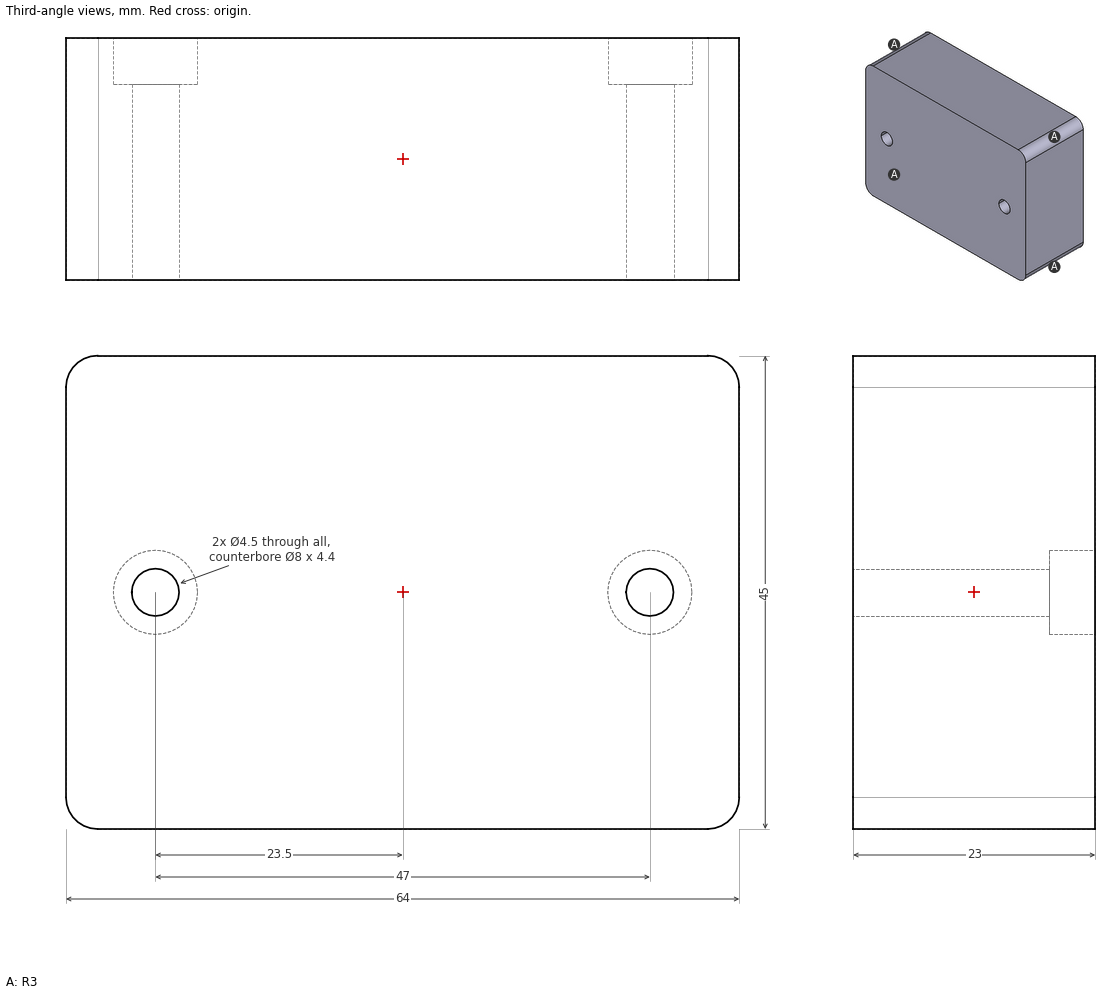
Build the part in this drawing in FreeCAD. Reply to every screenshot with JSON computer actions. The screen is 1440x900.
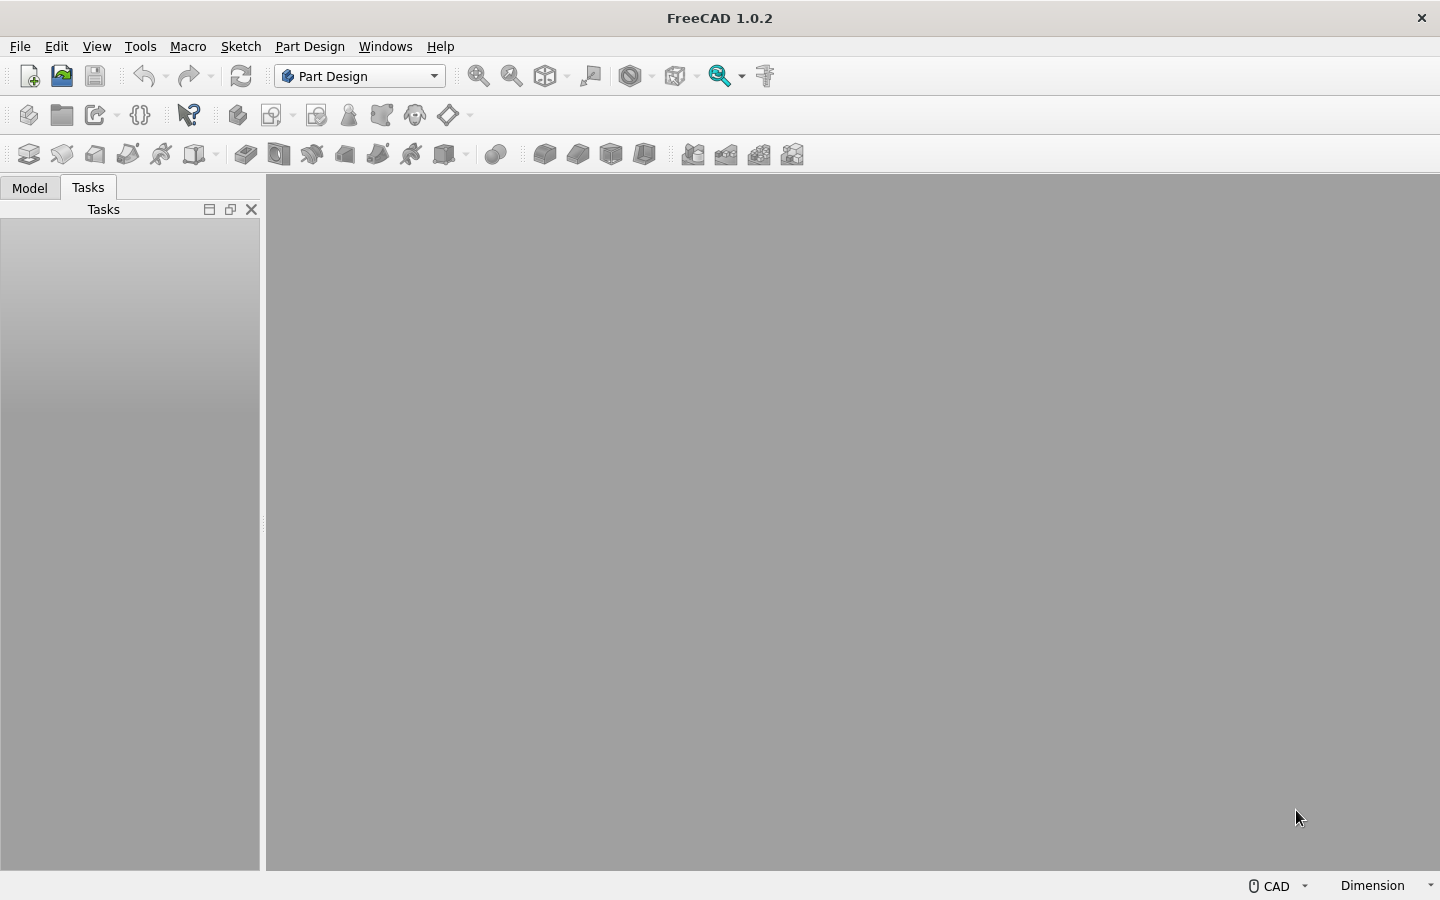
{"action": "left_click", "coordinate": [29, 76]}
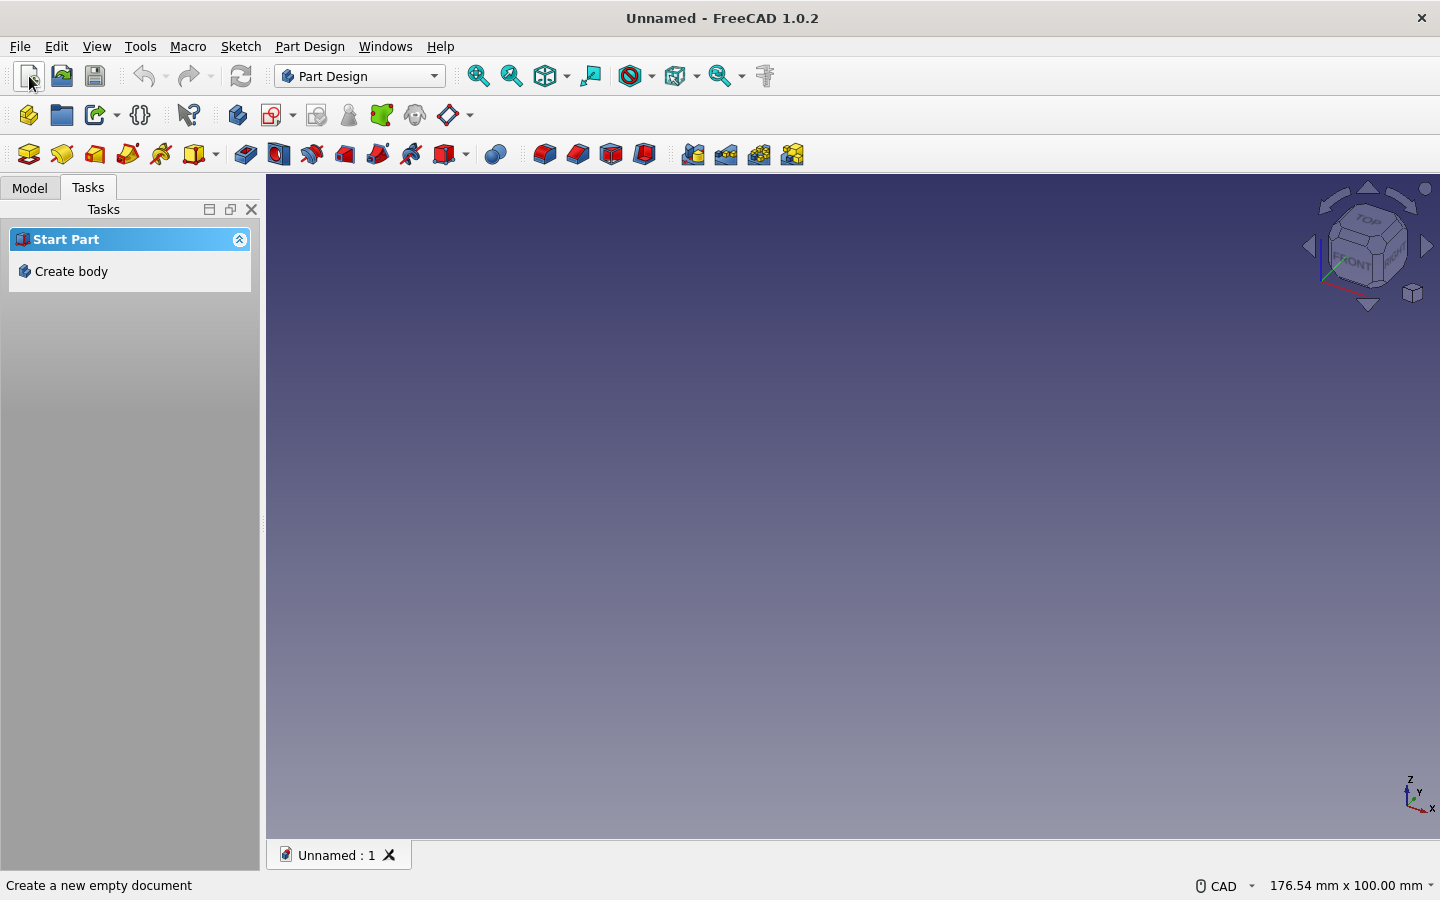
{"action": "left_click", "coordinate": [270, 116]}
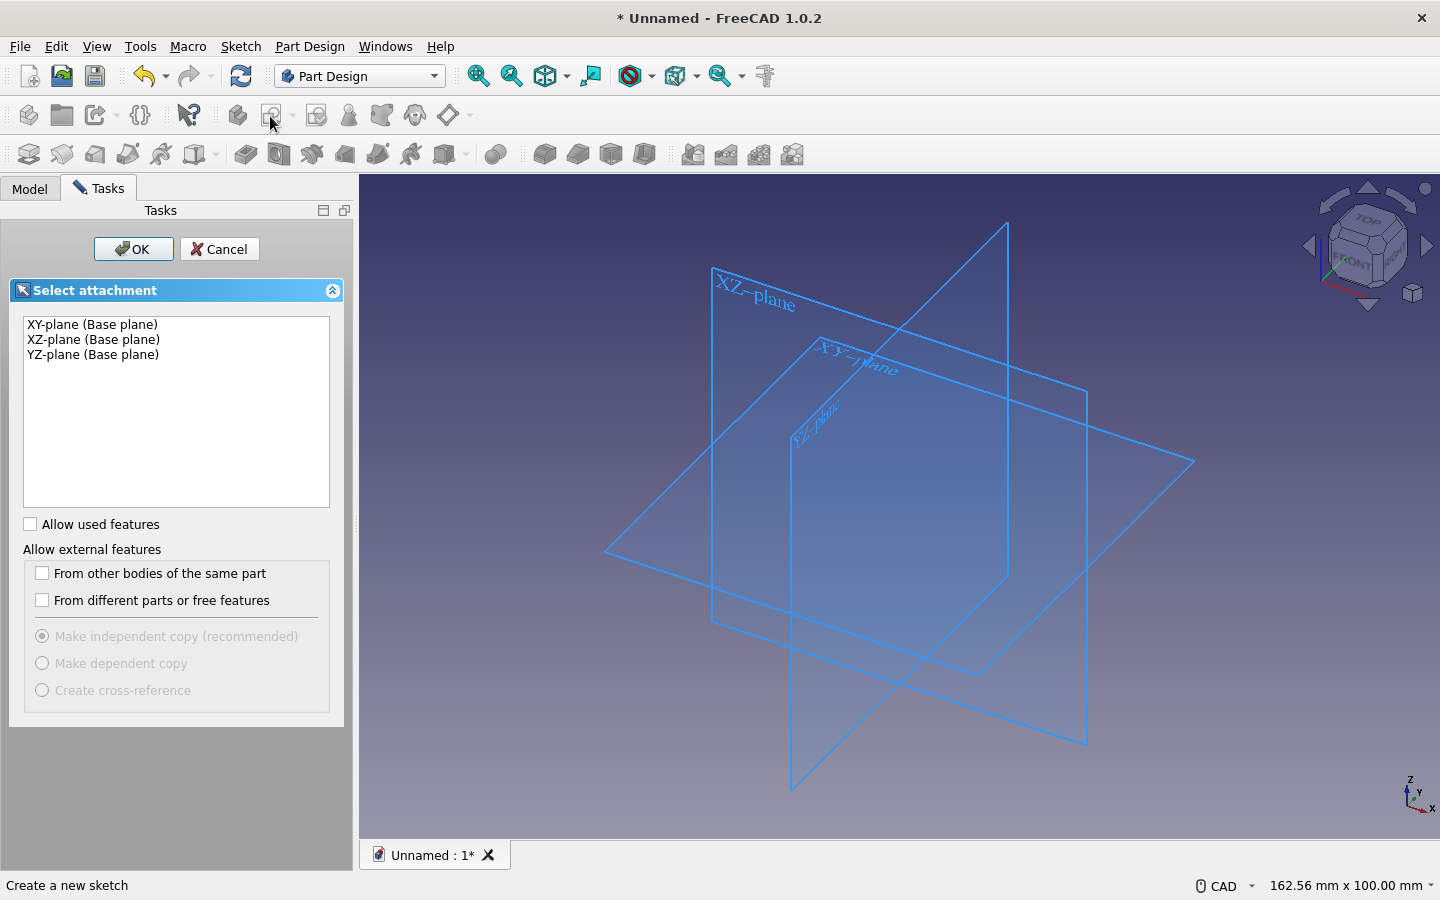
{"action": "left_click", "coordinate": [84, 340]}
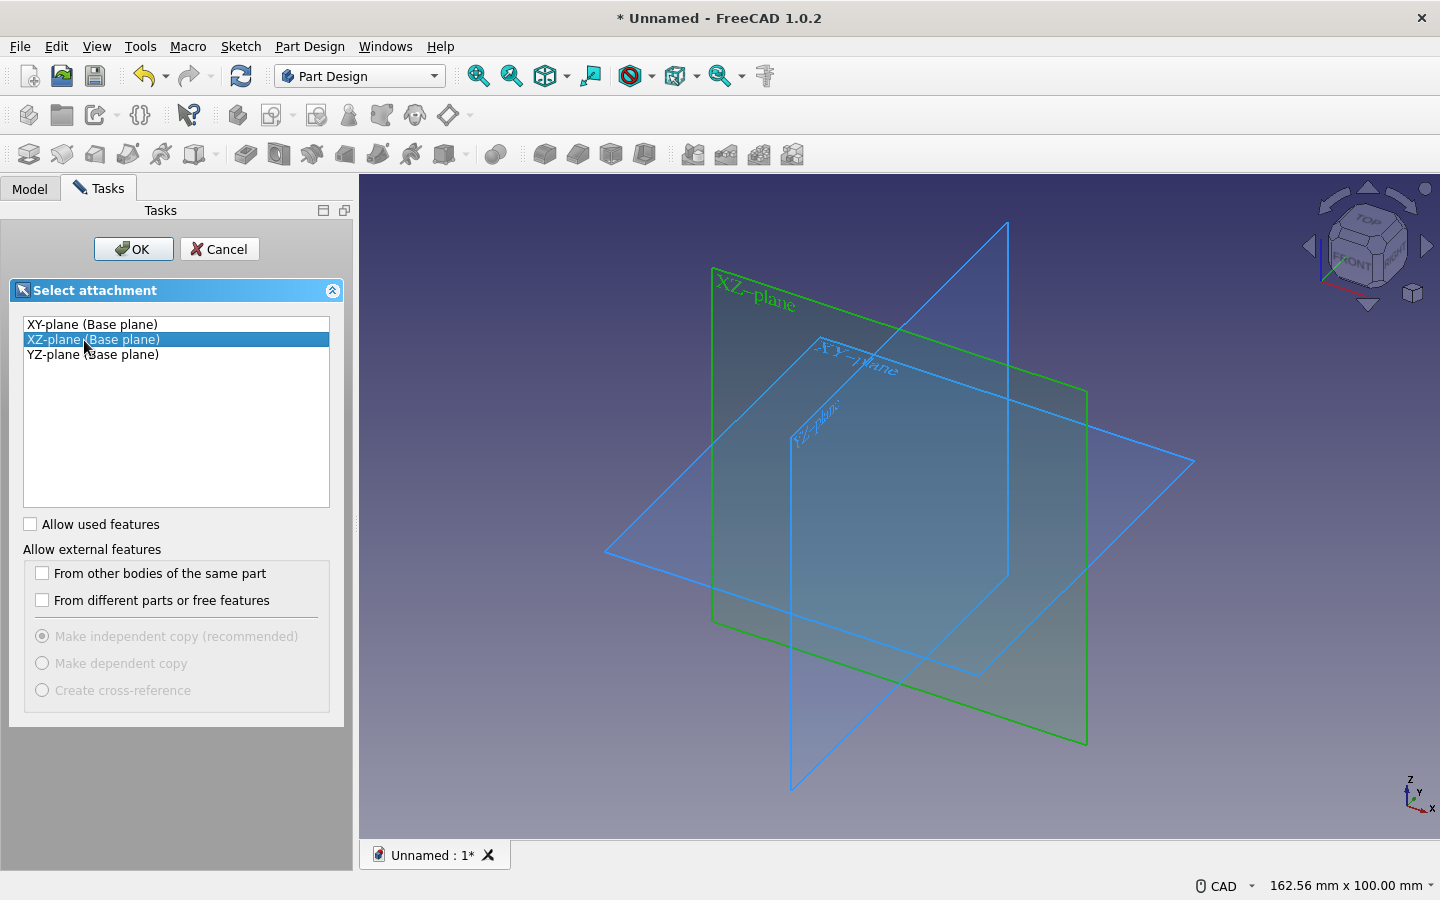
{"action": "left_click", "coordinate": [134, 249]}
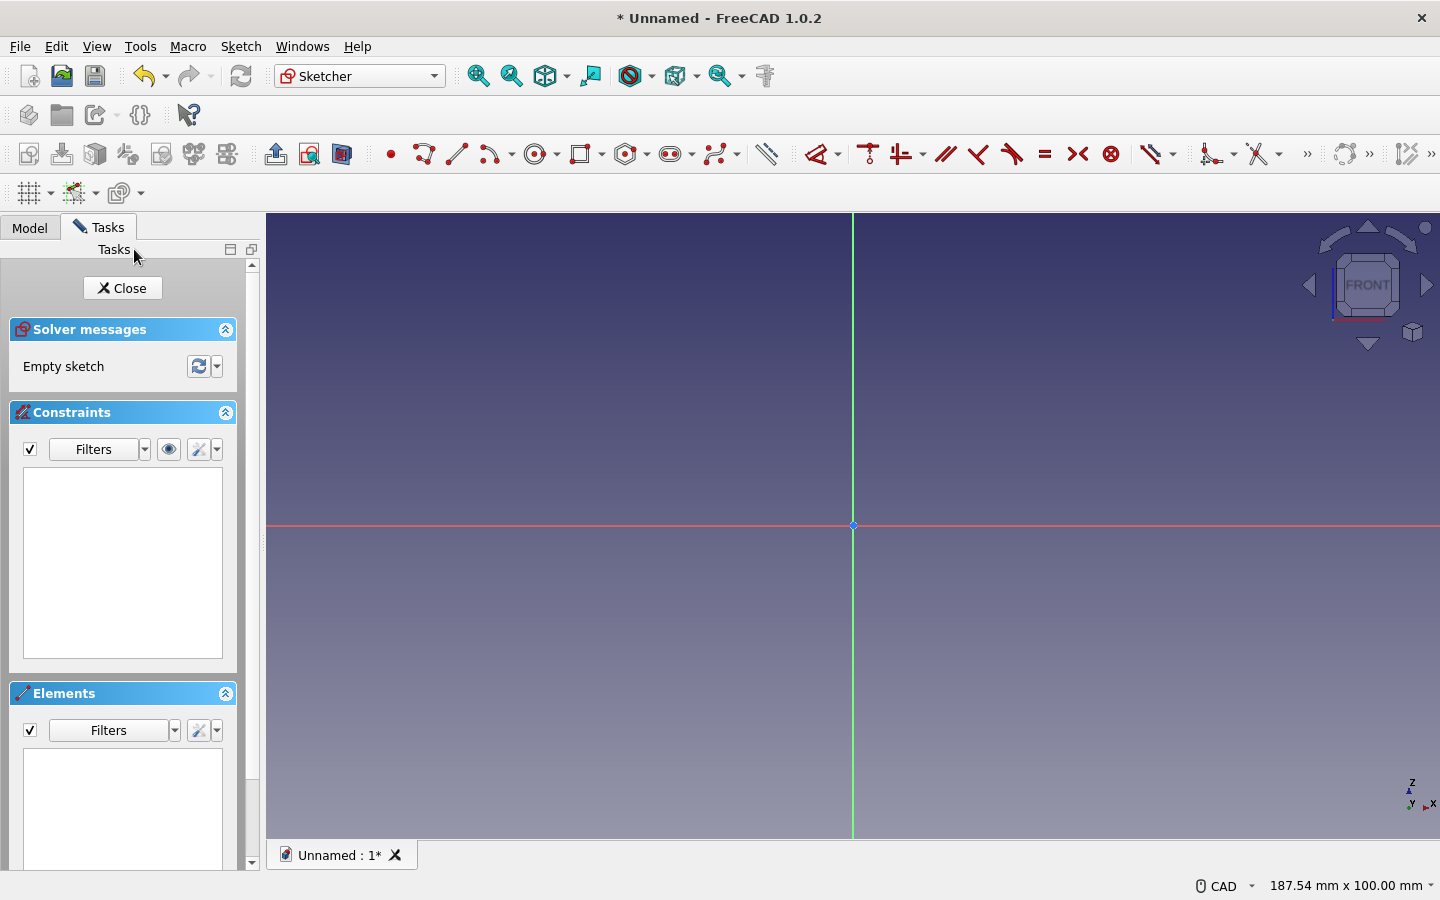
{"action": "scroll", "coordinate": [992, 526], "scroll_direction": "up", "scroll_amount": 2}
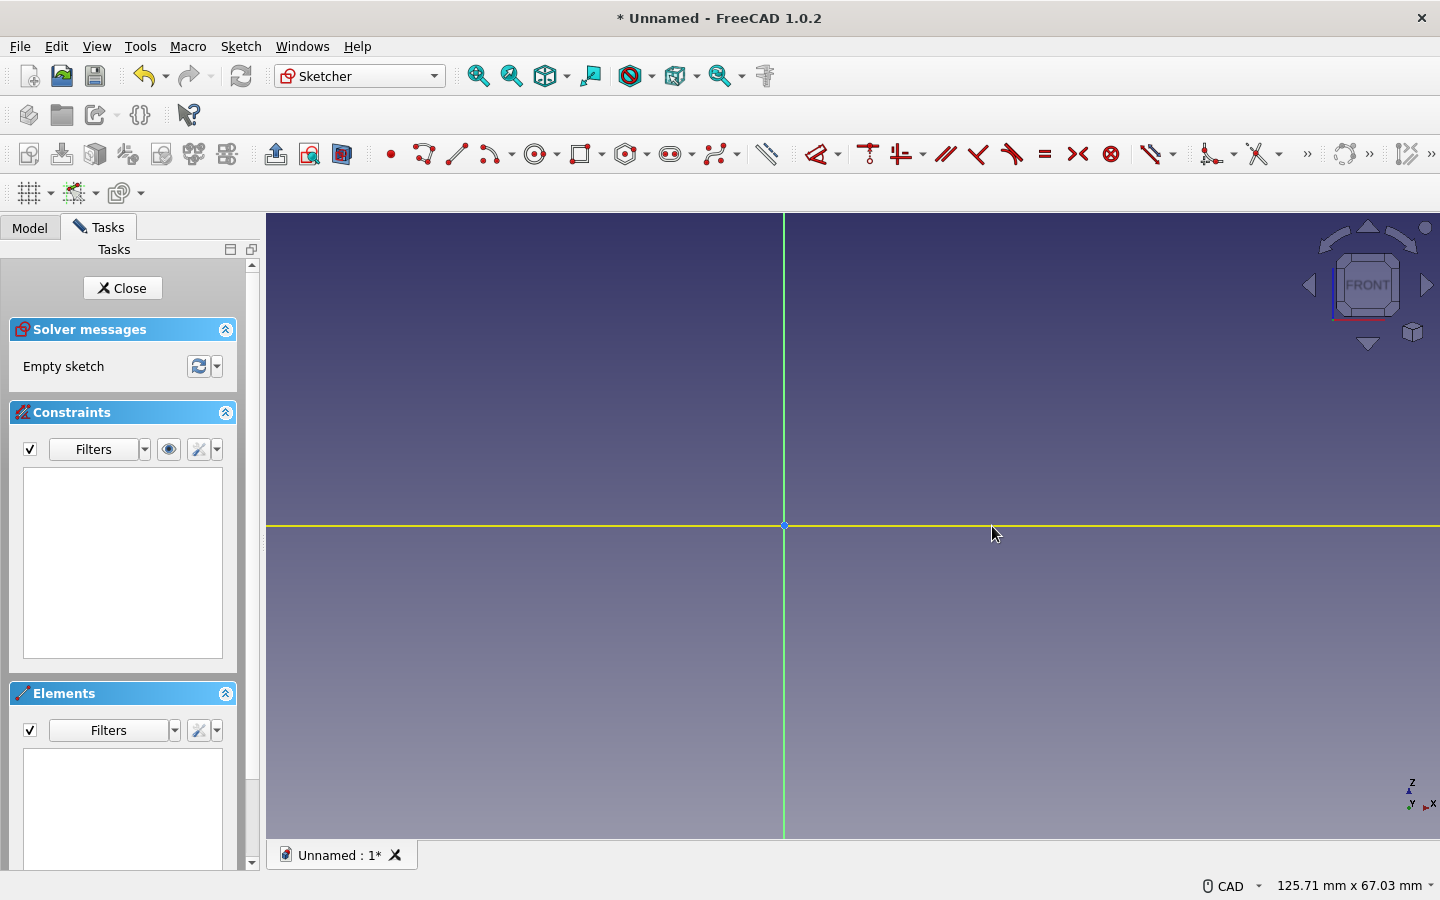
{"action": "left_click", "coordinate": [602, 154]}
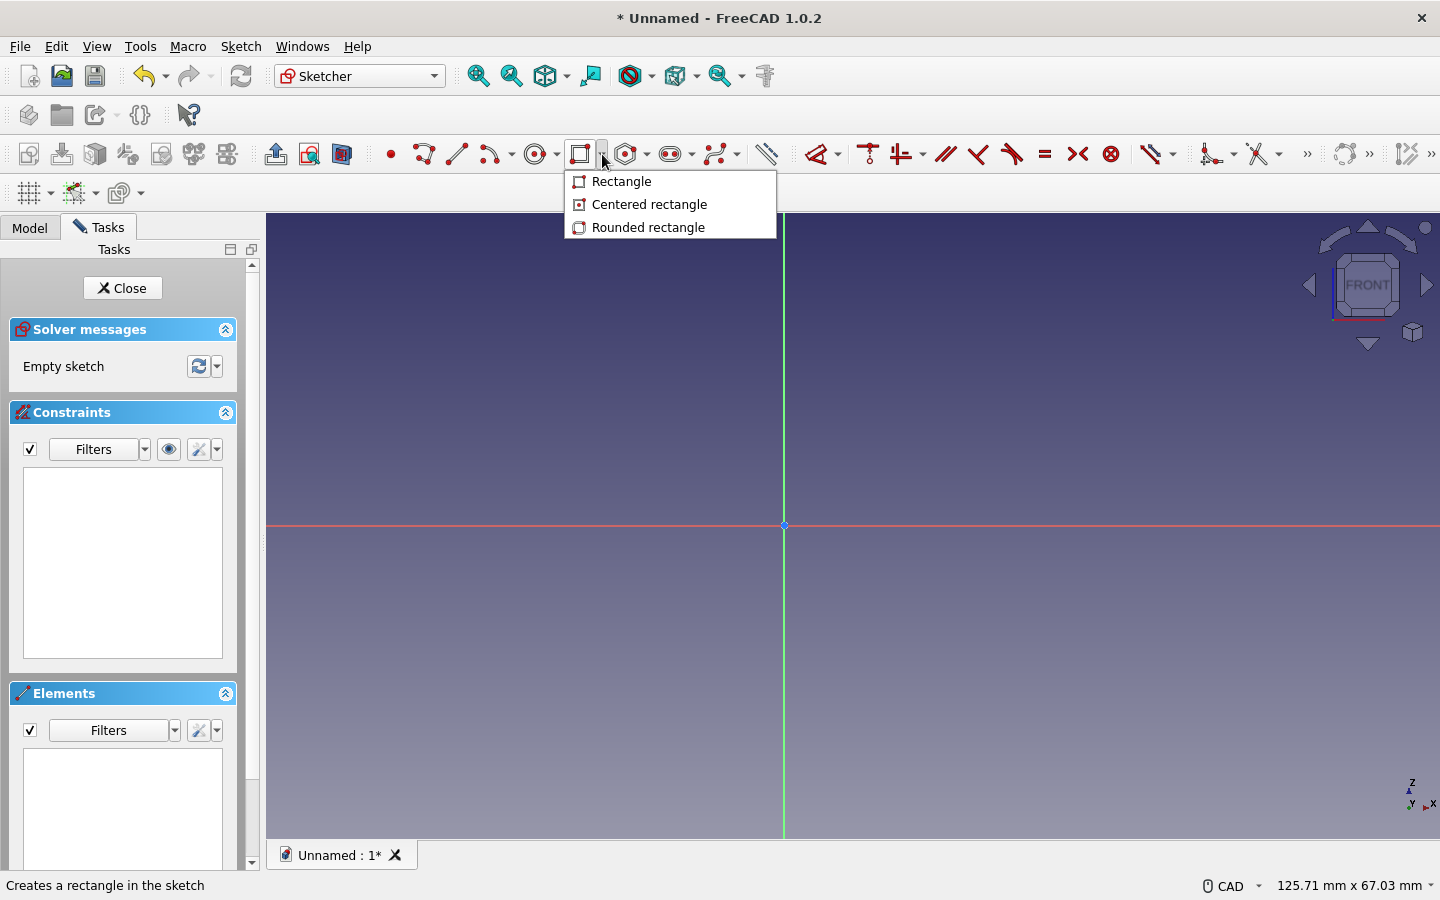
{"action": "left_click", "coordinate": [670, 204]}